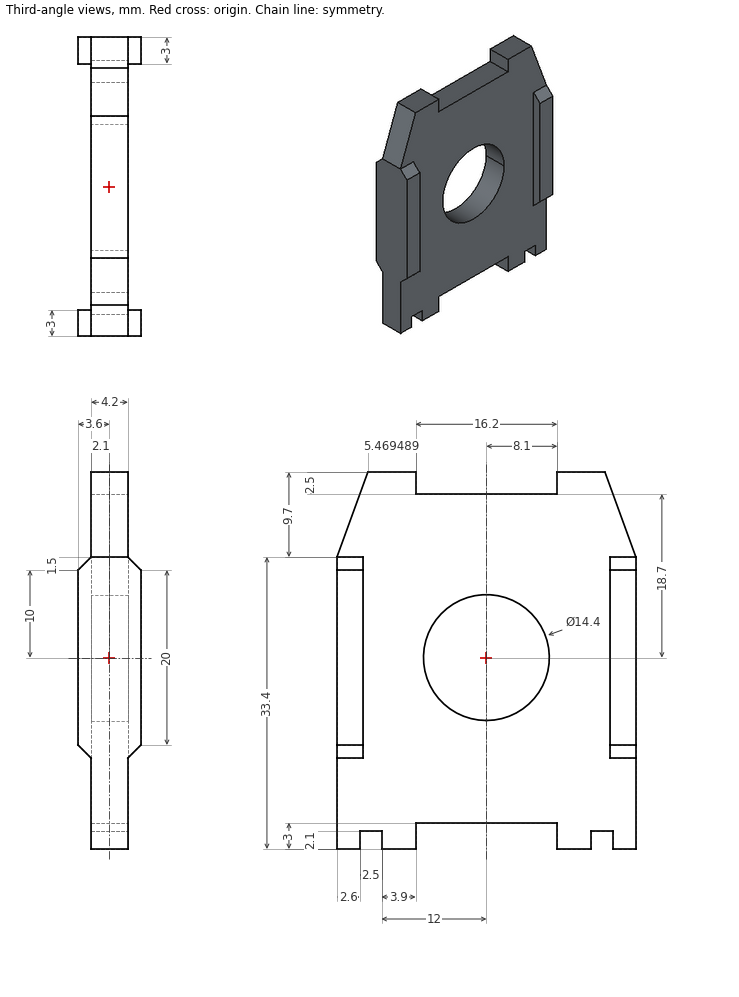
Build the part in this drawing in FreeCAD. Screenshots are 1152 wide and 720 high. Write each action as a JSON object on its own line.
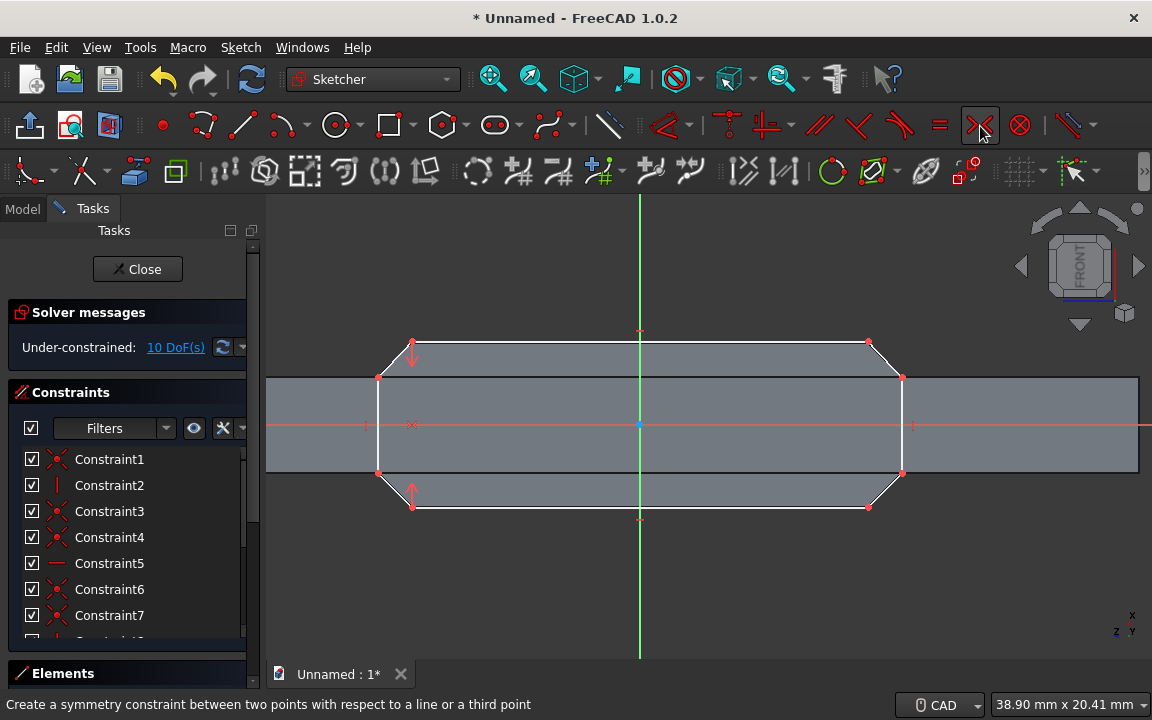
{"action": "left_click", "coordinate": [378, 378]}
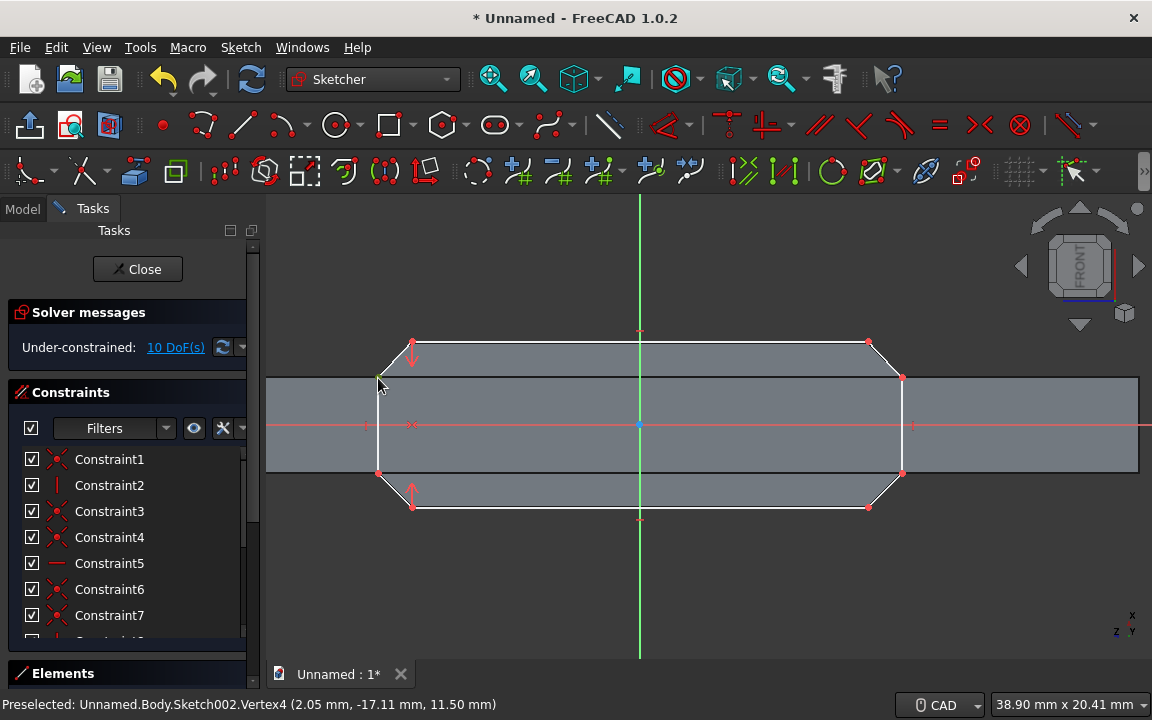
{"action": "left_click", "coordinate": [902, 378]}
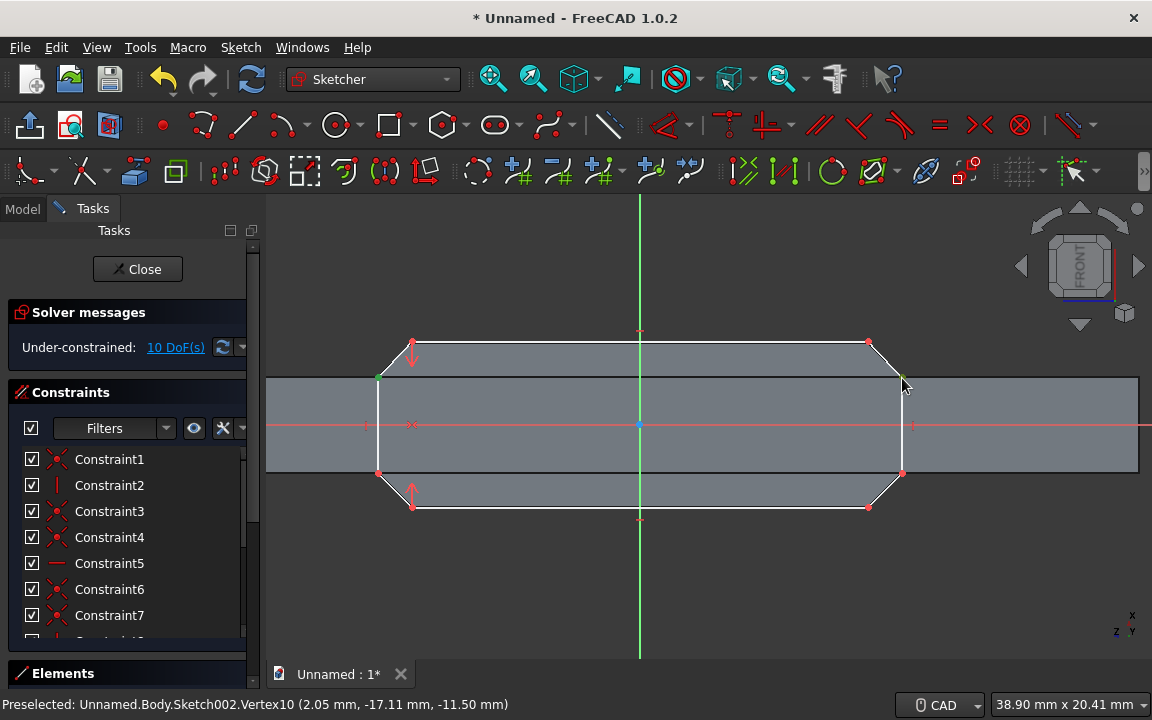
{"action": "left_click", "coordinate": [640, 602]}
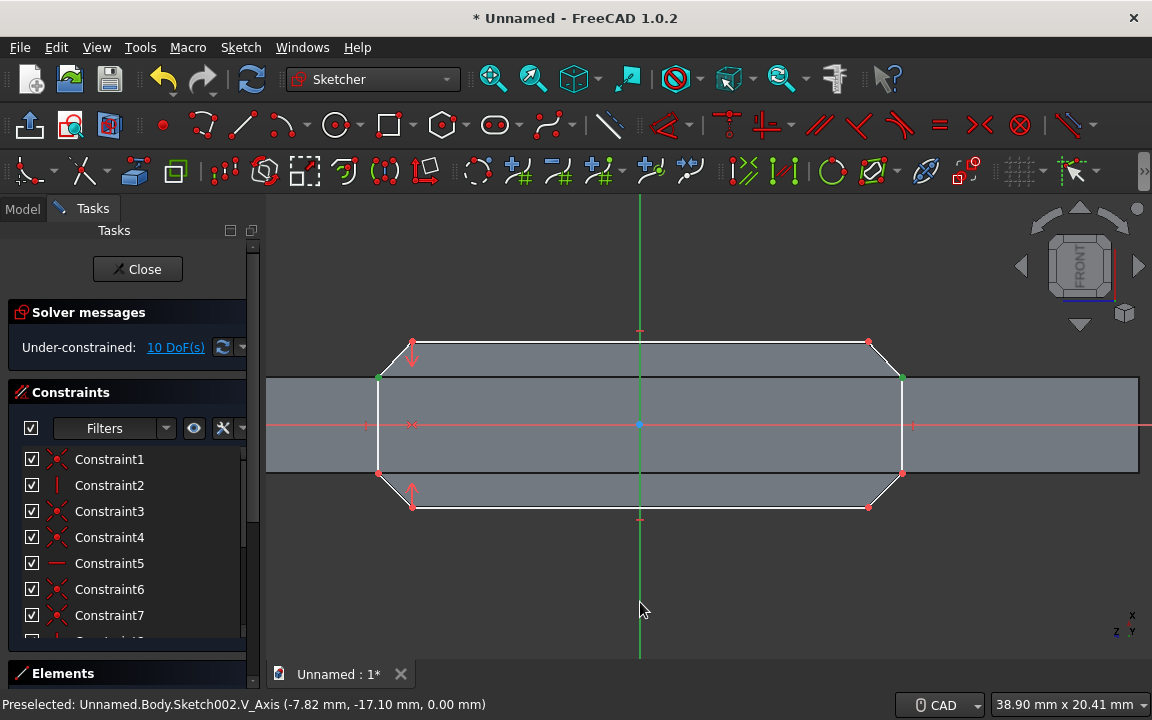
{"action": "left_click", "coordinate": [980, 126]}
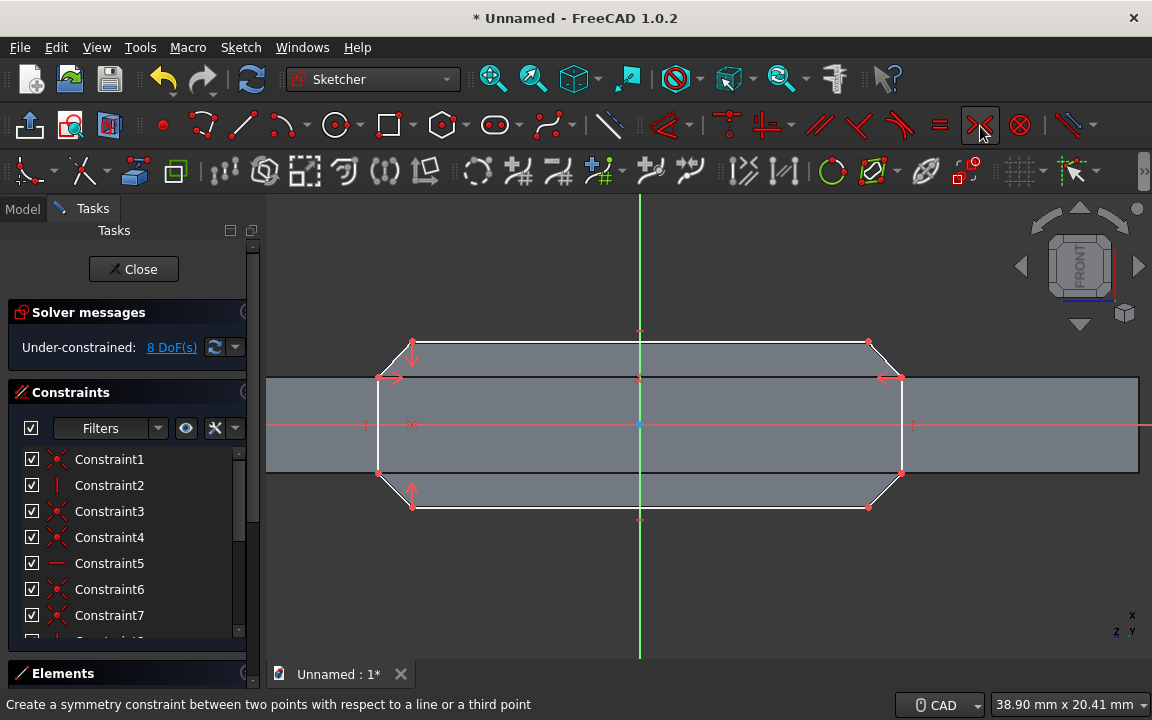
{"action": "left_click", "coordinate": [664, 126]}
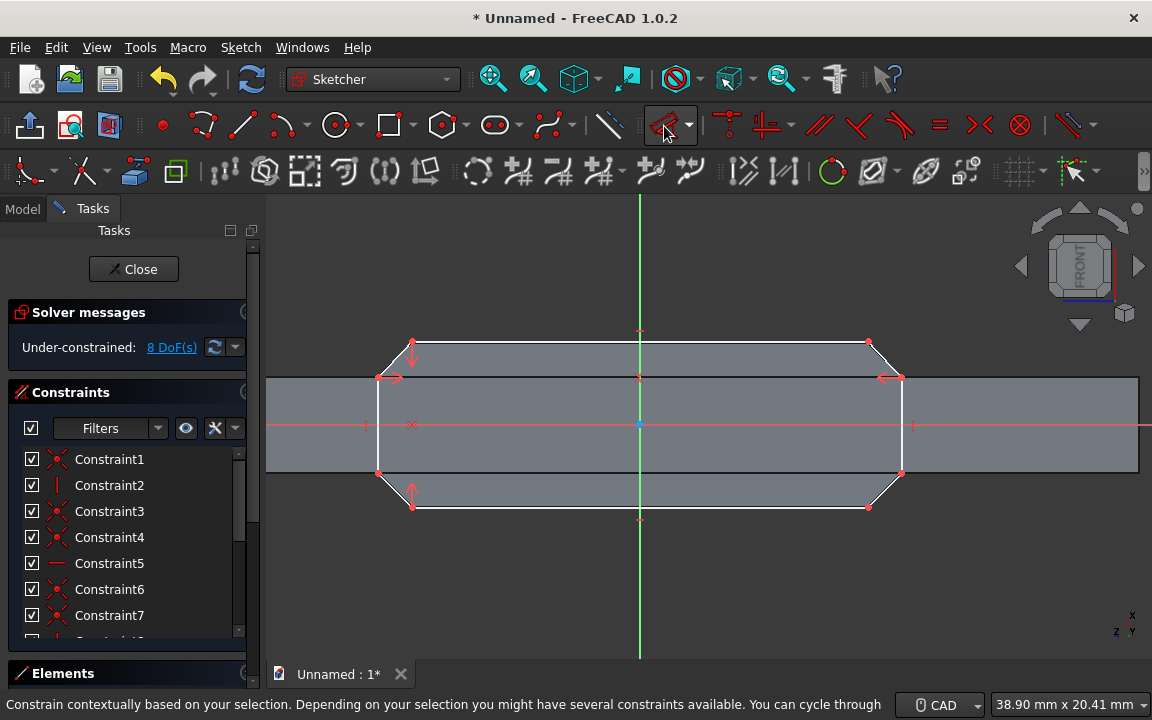
{"action": "left_click", "coordinate": [549, 342]}
{"action": "left_click", "coordinate": [535, 308]}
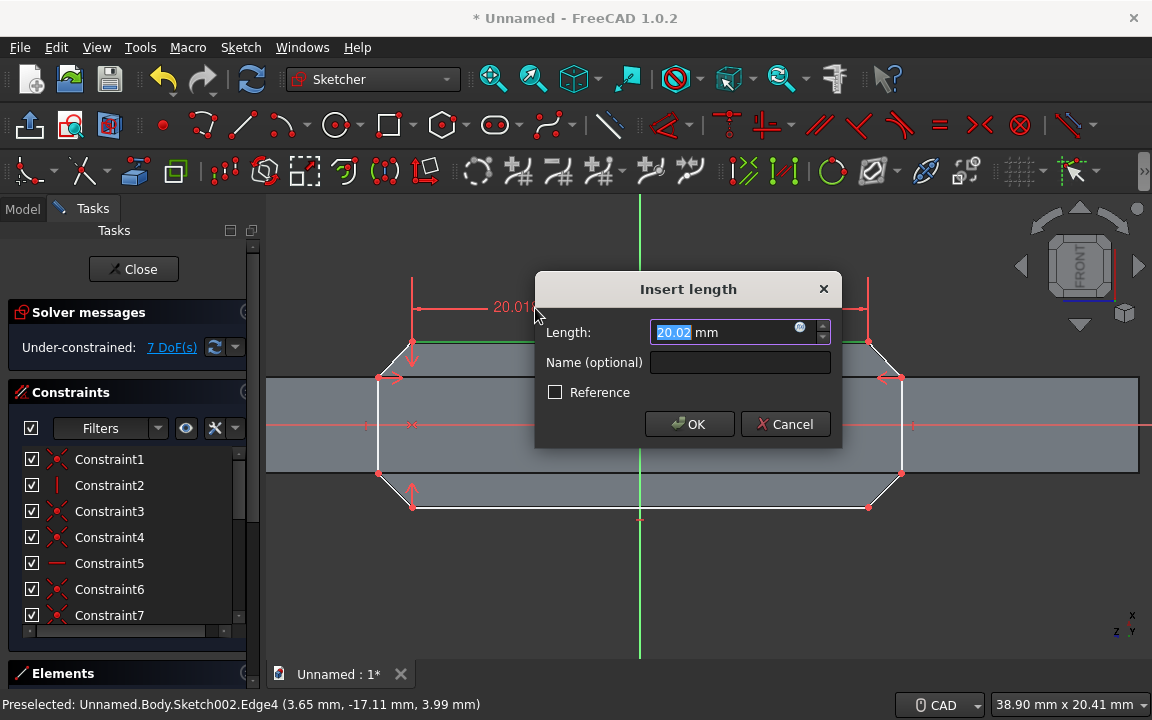
{"action": "type", "text": "20"}
{"action": "key", "text": "Return"}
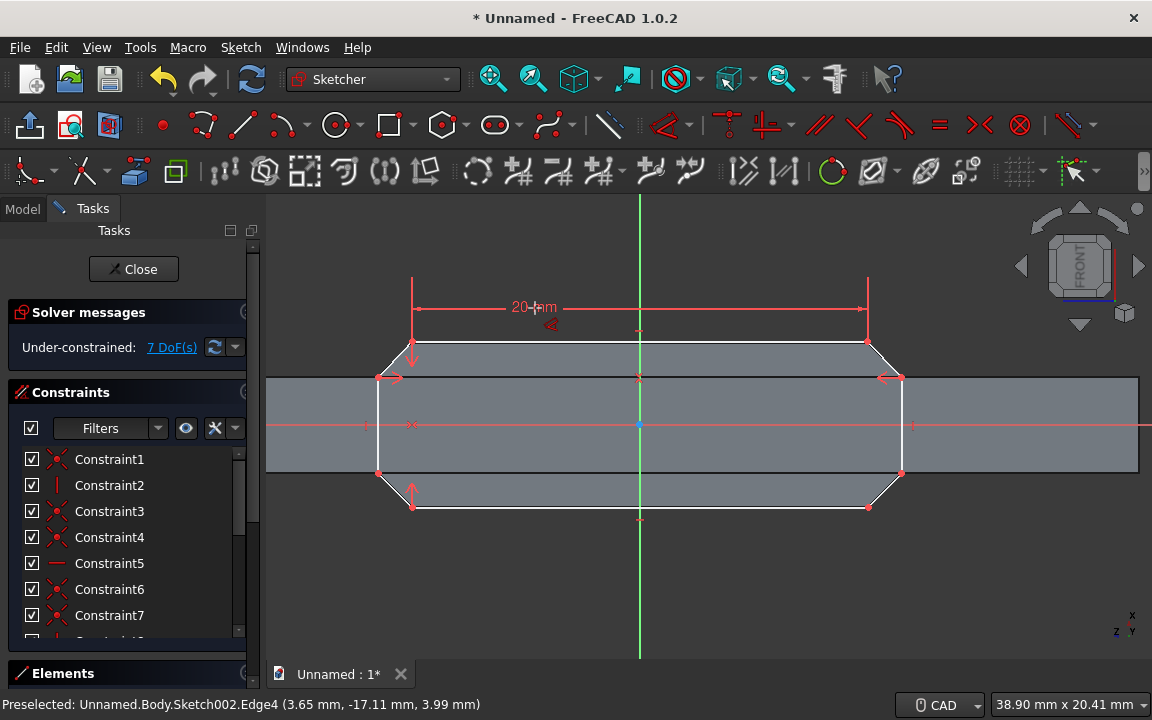
{"action": "left_click", "coordinate": [731, 508]}
{"action": "left_click", "coordinate": [535, 542]}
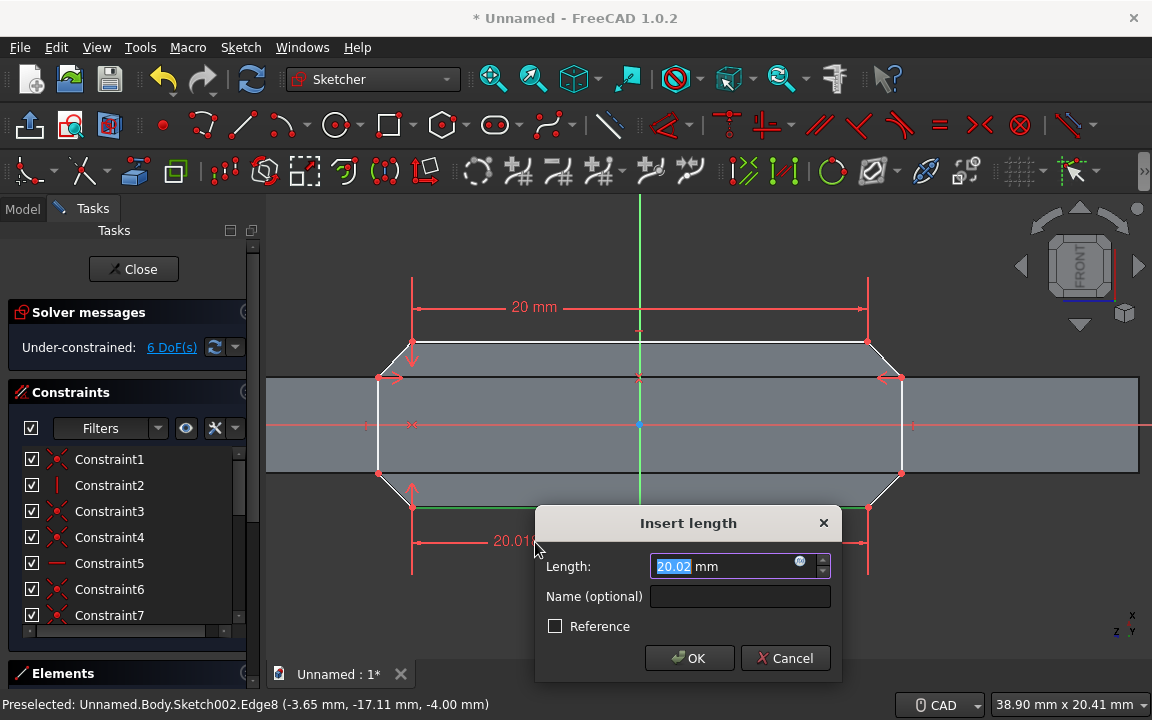
{"action": "type", "text": "20"}
{"action": "key", "text": "Return"}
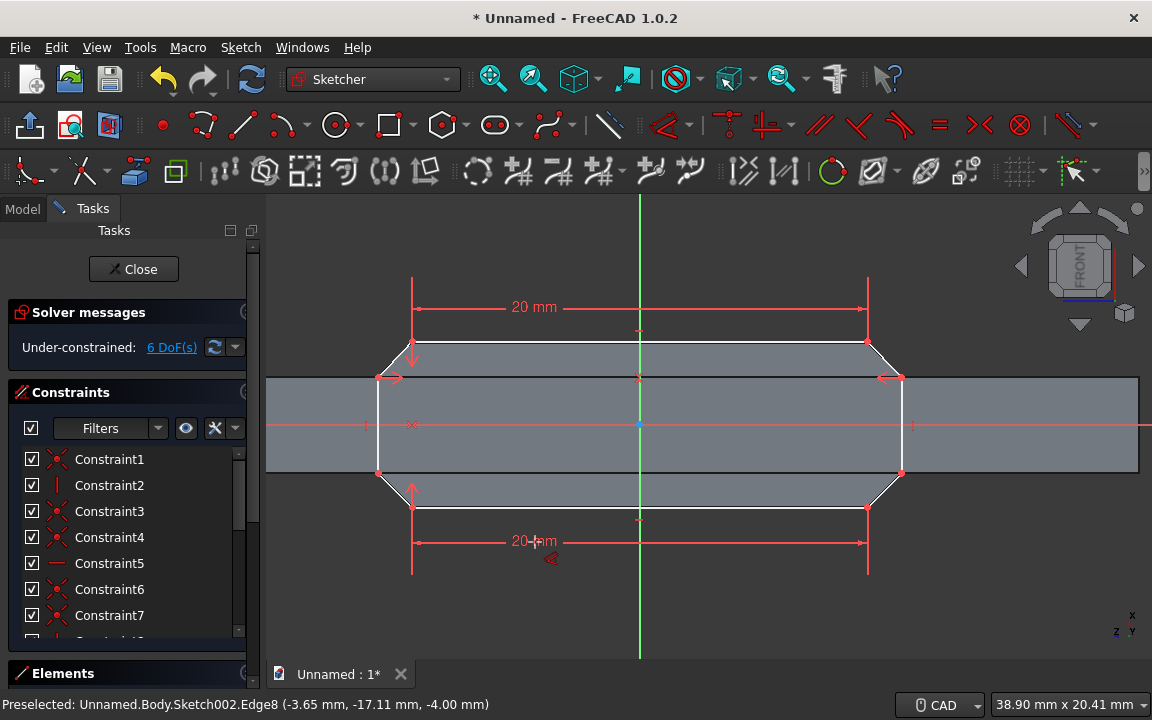
{"action": "left_click", "coordinate": [378, 445]}
{"action": "left_click", "coordinate": [344, 404]}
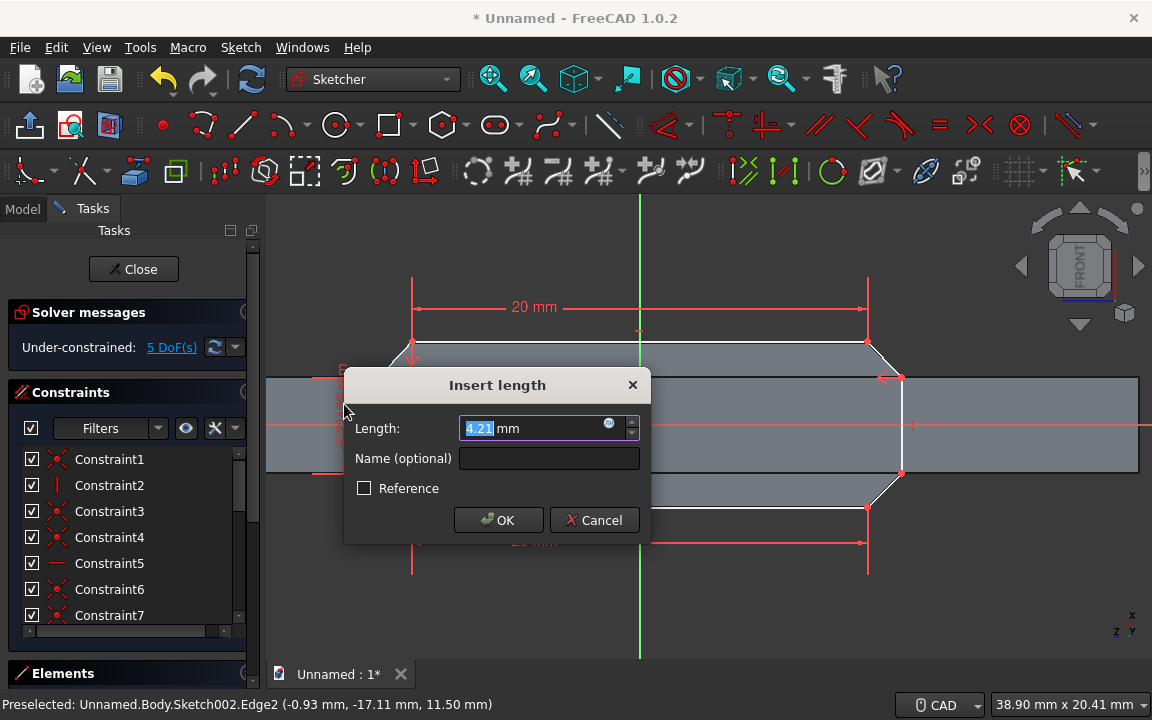
{"action": "type", "text": "4.2"}
{"action": "key", "text": "Return"}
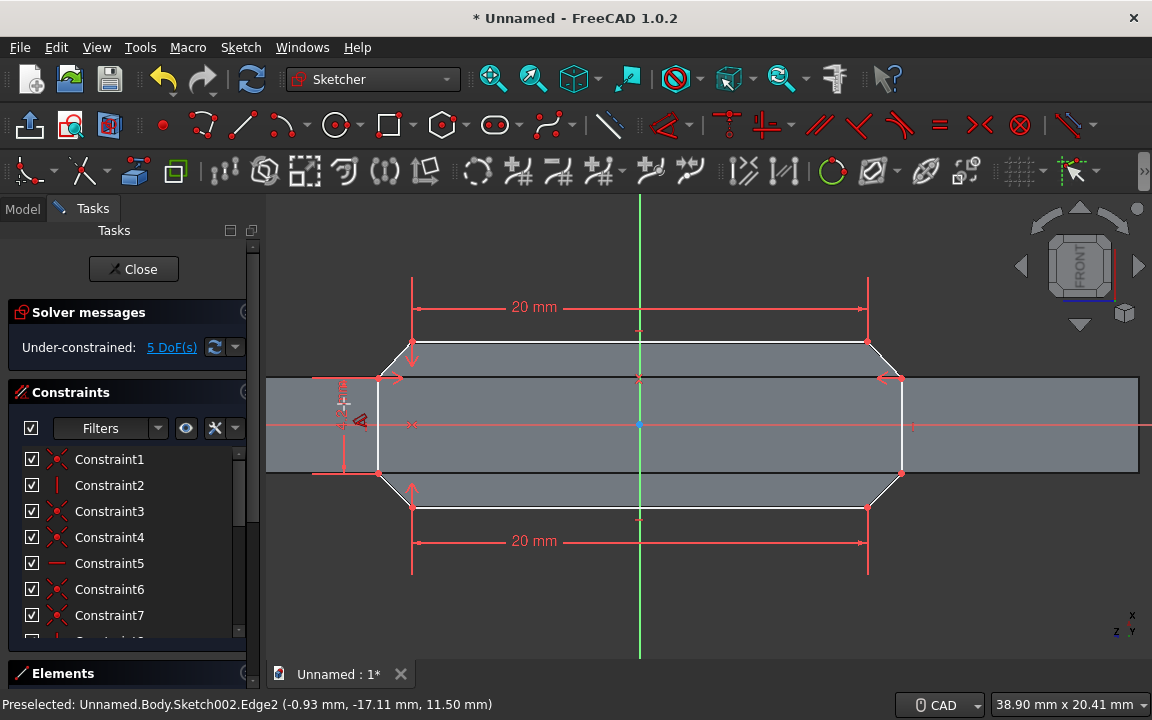
{"action": "left_click", "coordinate": [902, 407]}
{"action": "left_click", "coordinate": [936, 404]}